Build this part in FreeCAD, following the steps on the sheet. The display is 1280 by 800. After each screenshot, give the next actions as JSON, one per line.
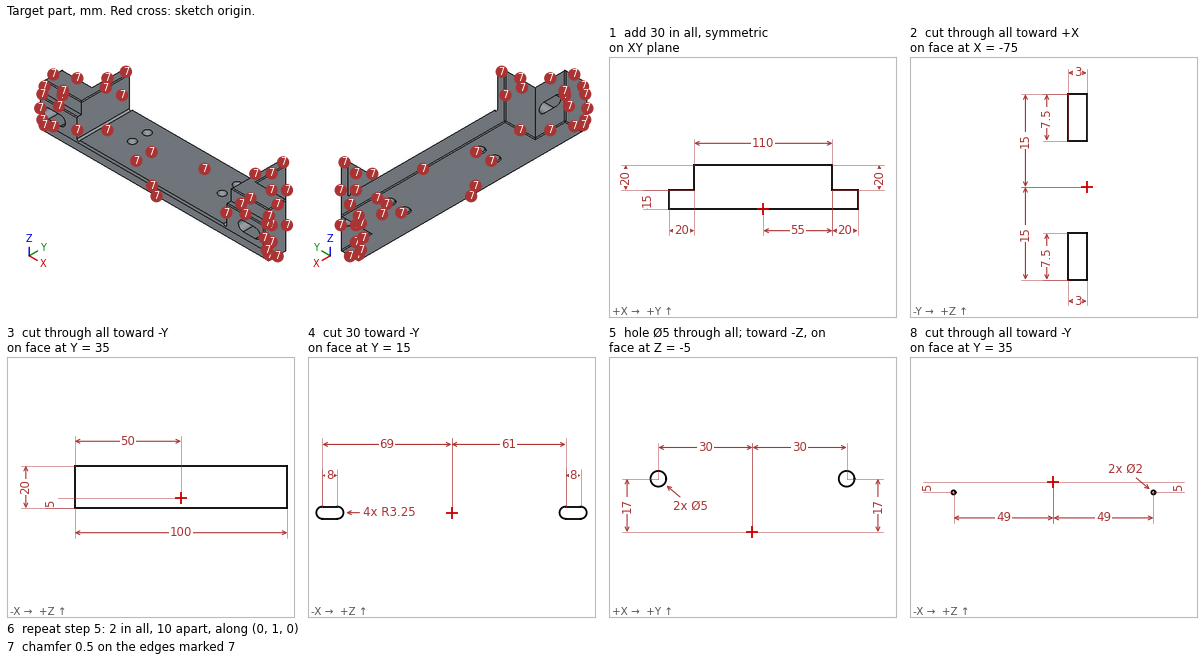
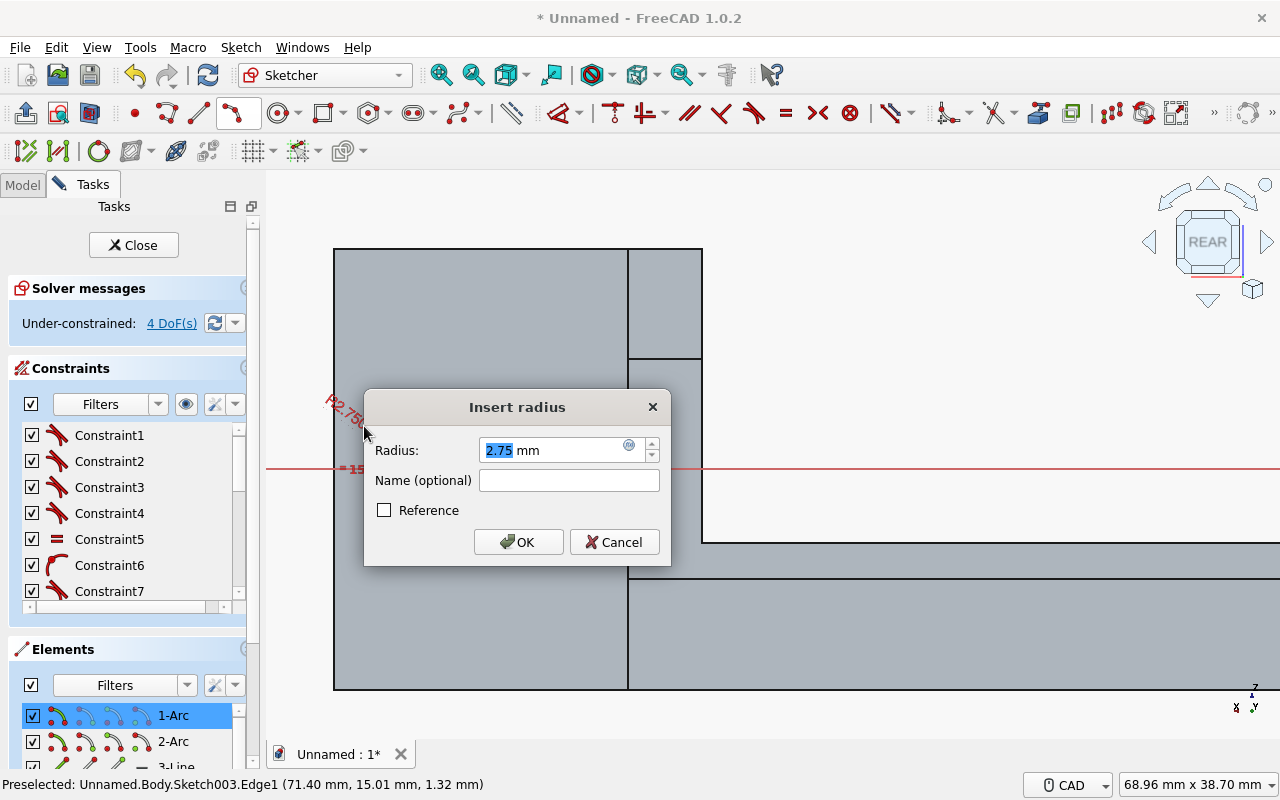
{"action": "type", "text": "3.25"}
{"action": "key", "text": "Return"}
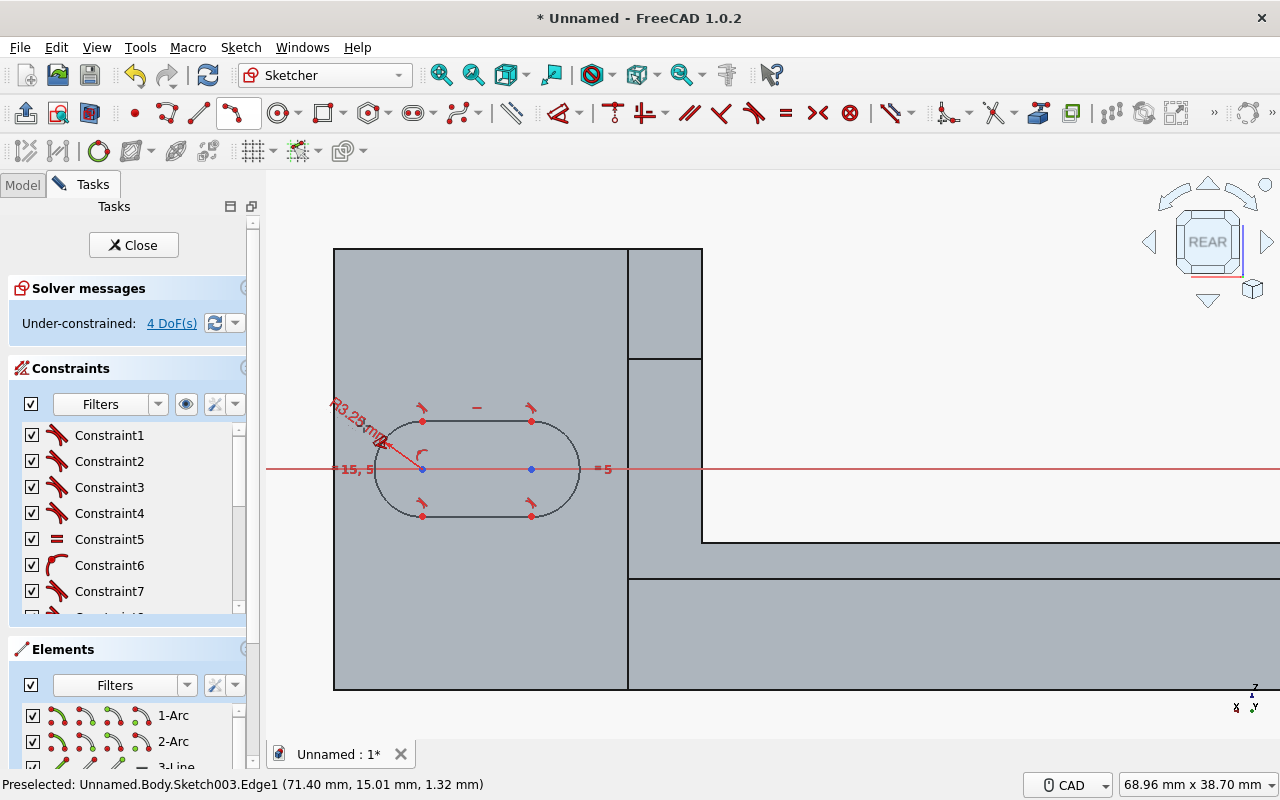
{"action": "left_click", "coordinate": [455, 421]}
{"action": "left_click", "coordinate": [477, 387]}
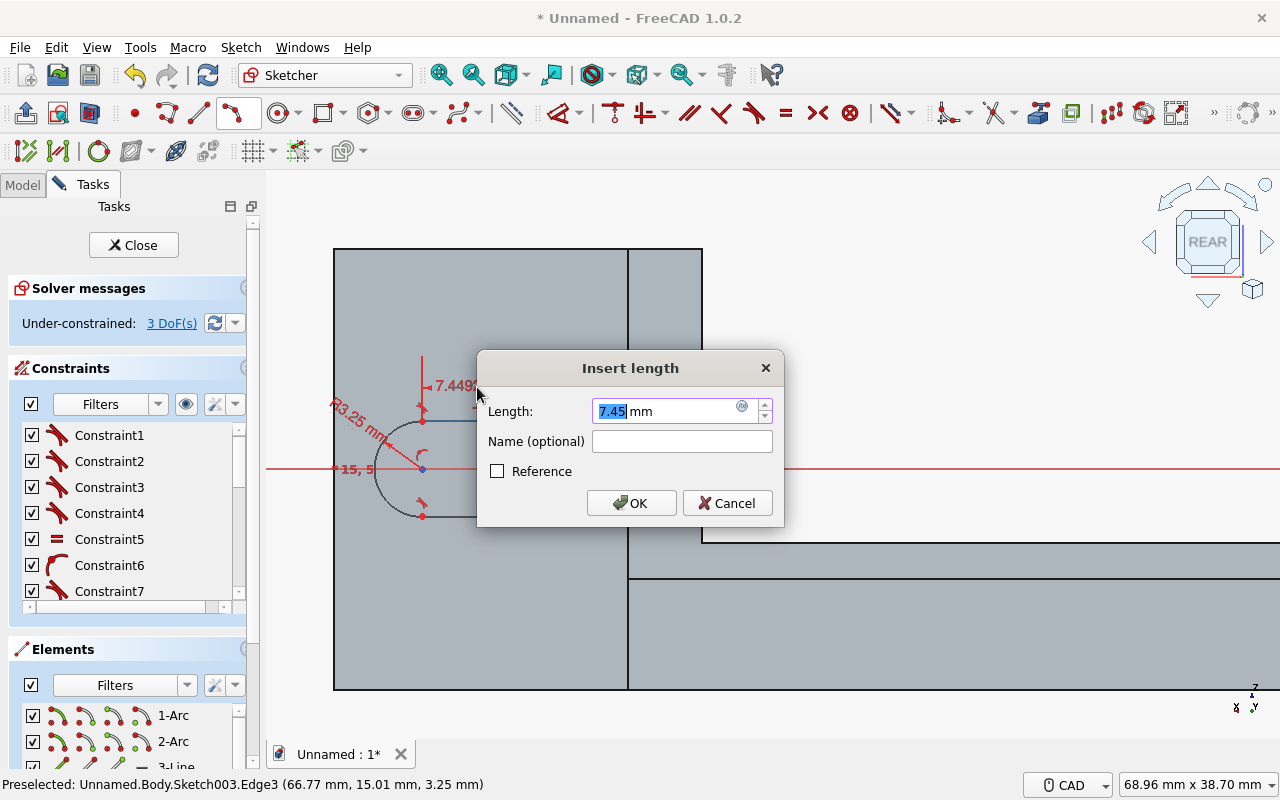
{"action": "type", "text": "8"}
{"action": "key", "text": "Return"}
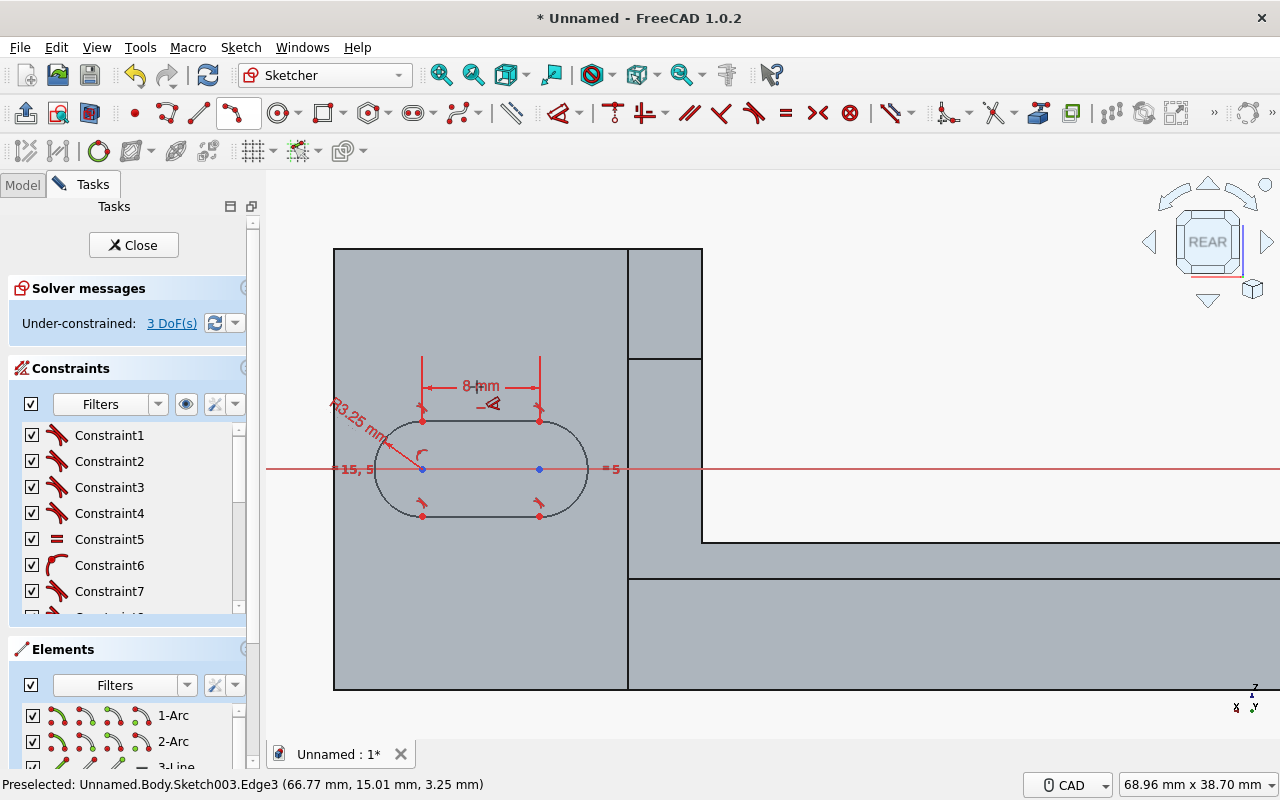
{"action": "scroll", "coordinate": [389, 448], "scroll_direction": "down", "scroll_amount": 6}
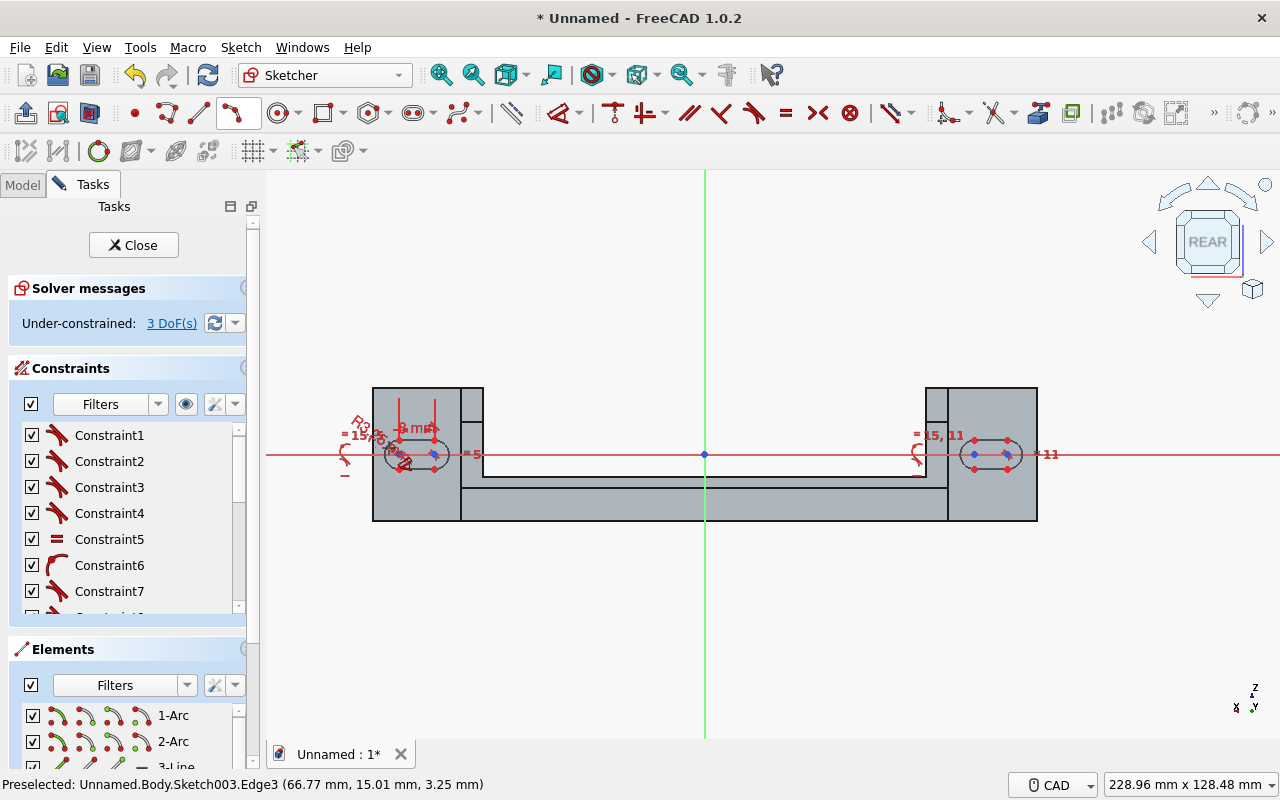
{"action": "scroll", "coordinate": [985, 440], "scroll_direction": "up", "scroll_amount": 2}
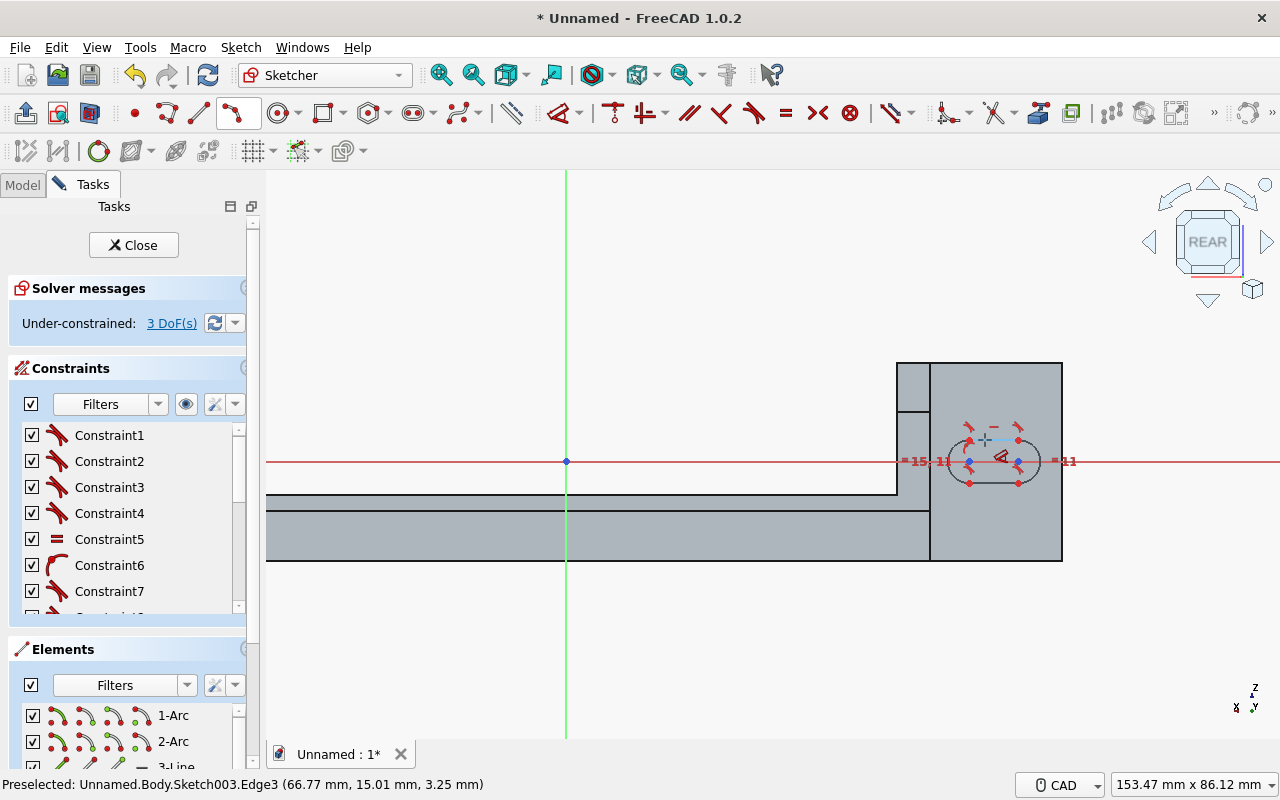
{"action": "left_click", "coordinate": [984, 440]}
{"action": "left_click", "coordinate": [994, 406]}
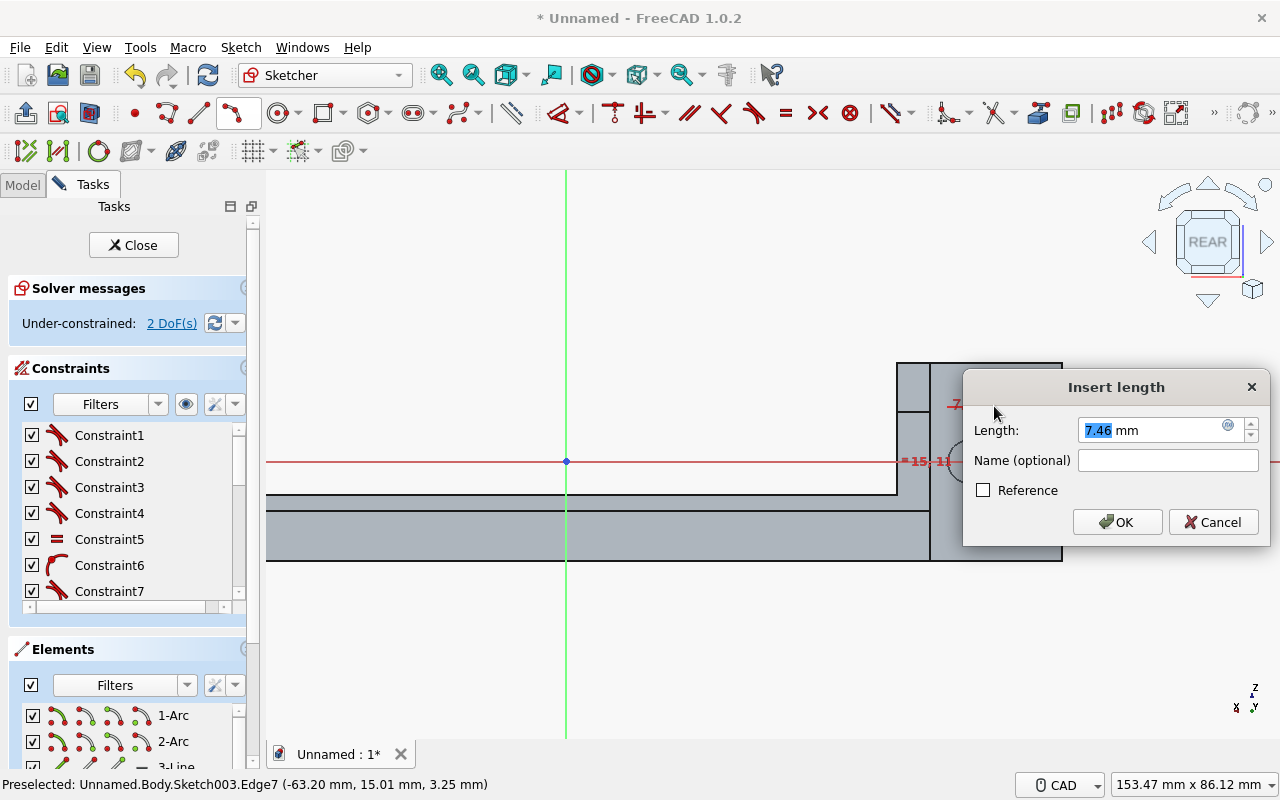
{"action": "type", "text": "8"}
{"action": "key", "text": "Return"}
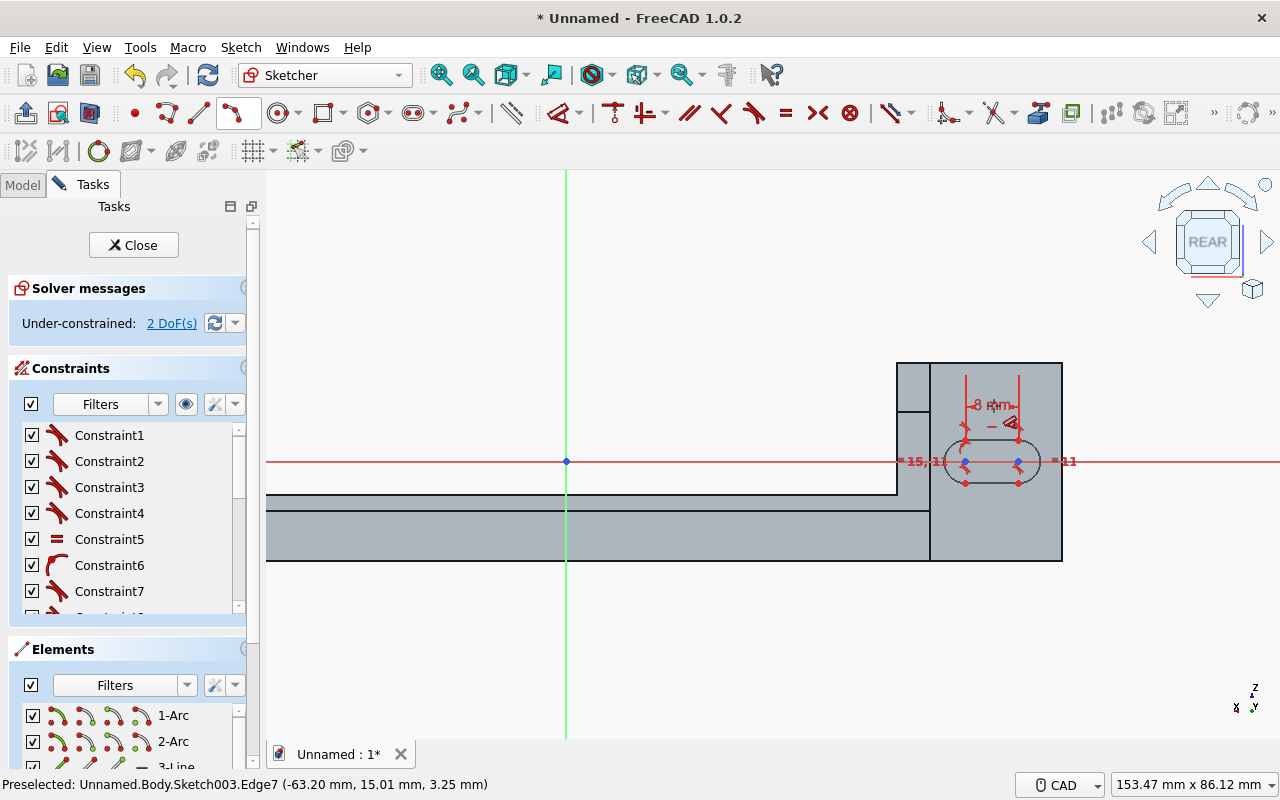
{"action": "scroll", "coordinate": [985, 440], "scroll_direction": "down", "scroll_amount": 2}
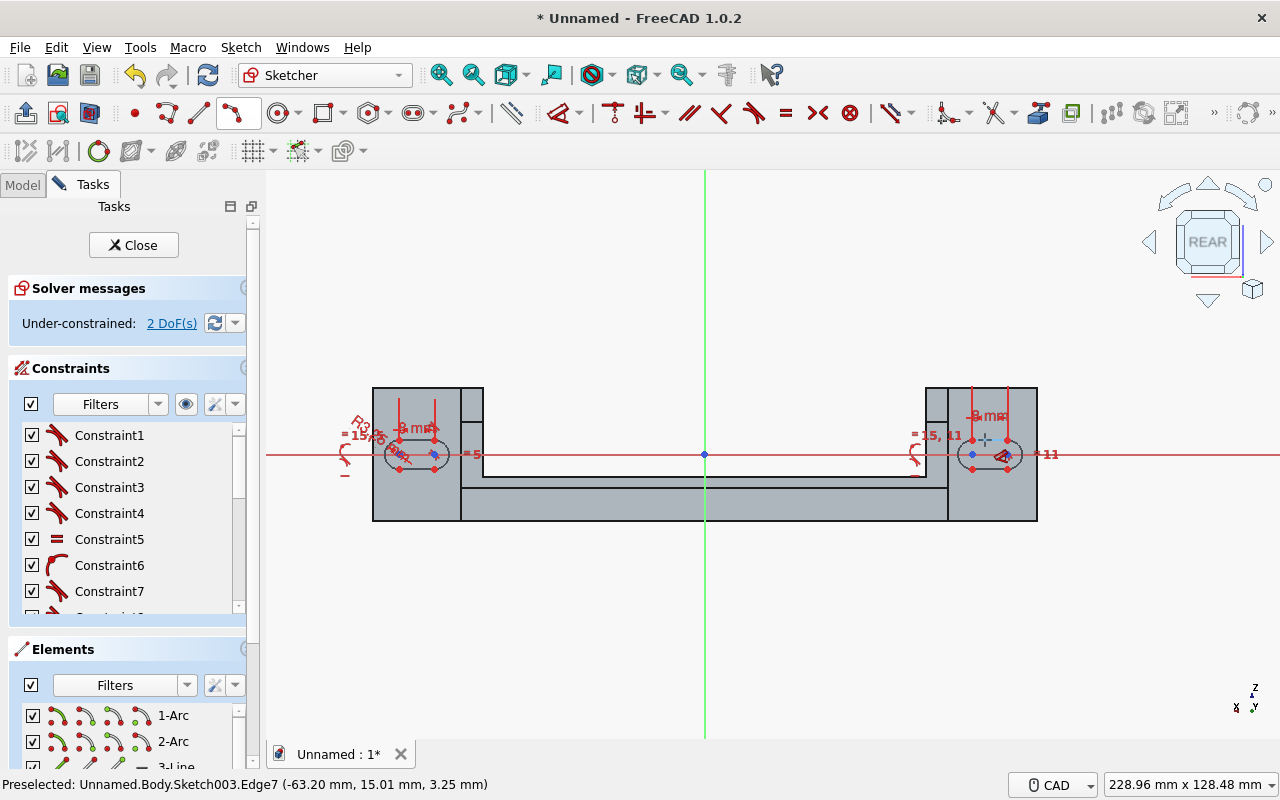
{"action": "left_click", "coordinate": [399, 440]}
{"action": "left_click", "coordinate": [552, 406]}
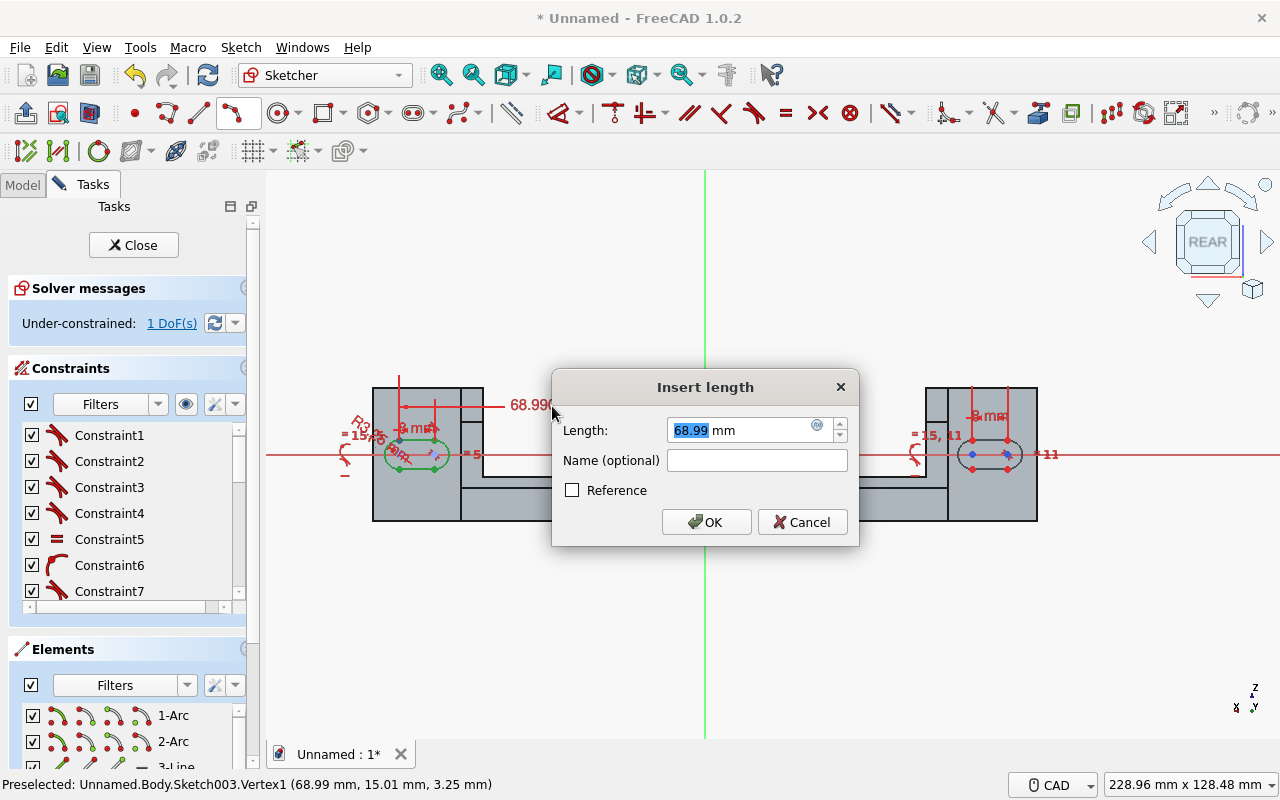
{"action": "type", "text": "69"}
{"action": "key", "text": "Return"}